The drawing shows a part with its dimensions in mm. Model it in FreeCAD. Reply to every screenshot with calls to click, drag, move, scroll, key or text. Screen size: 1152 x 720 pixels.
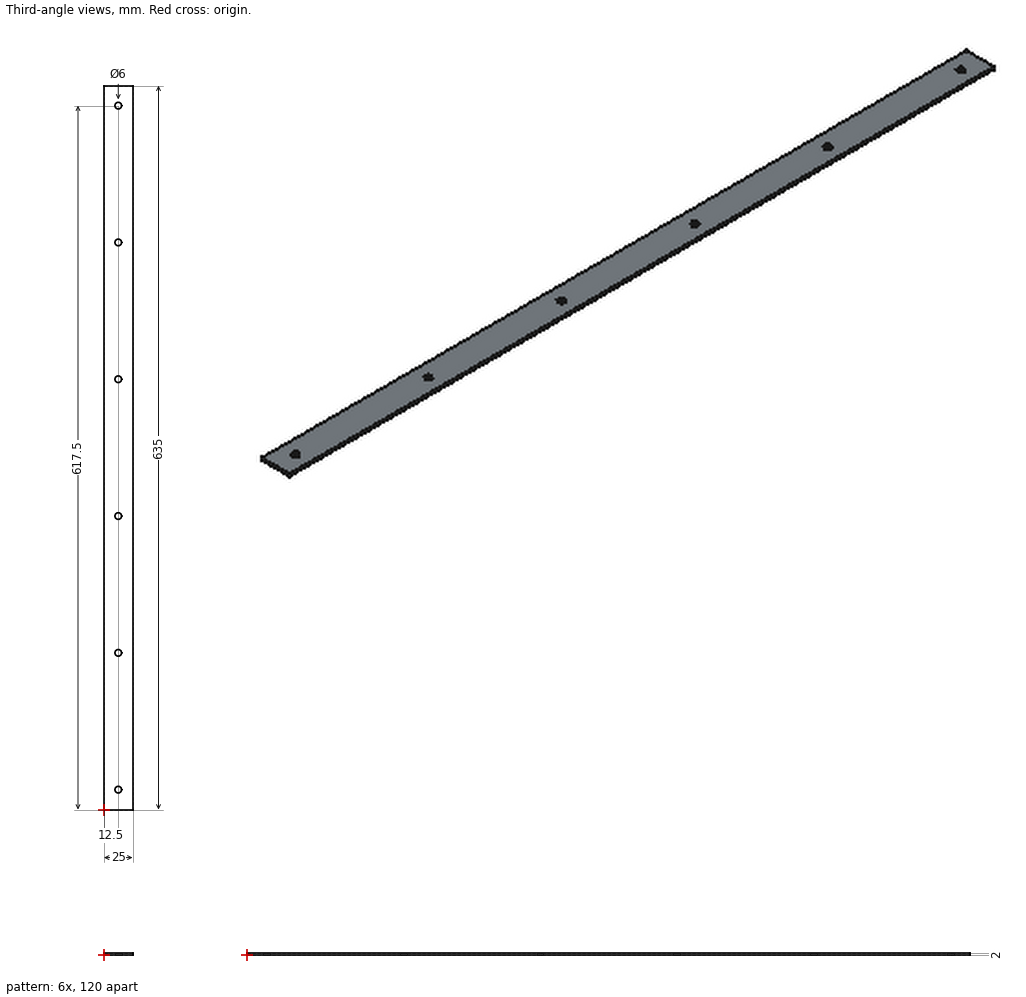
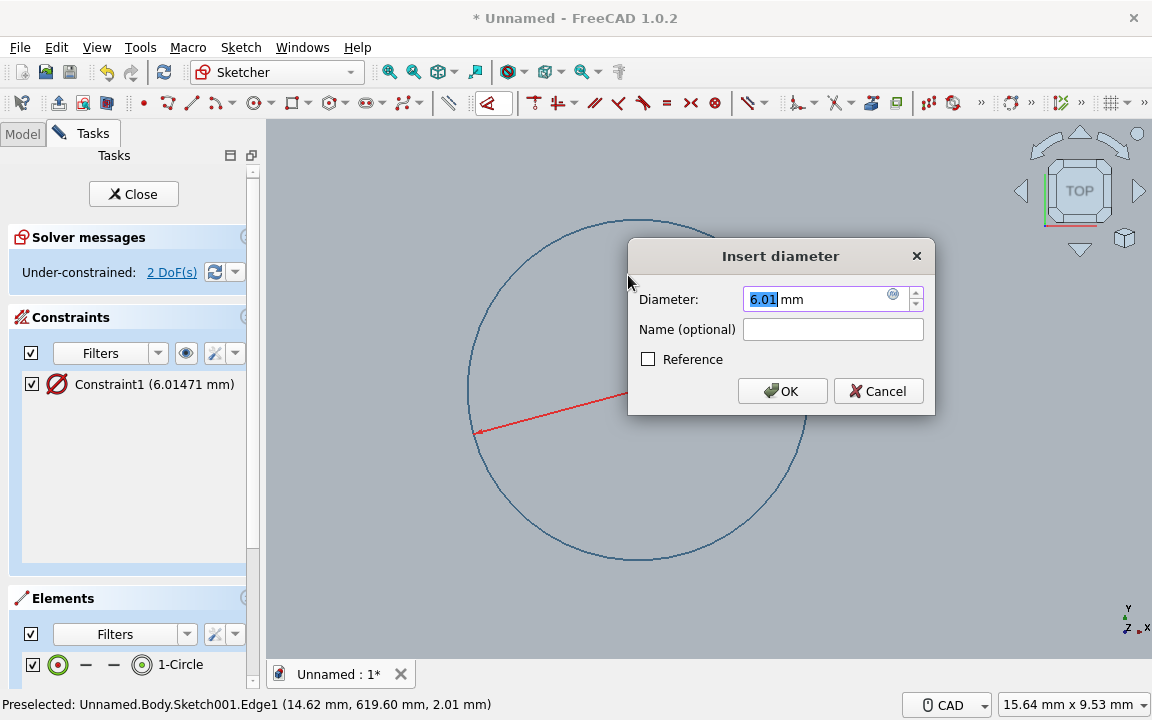
text(6)
key(Return)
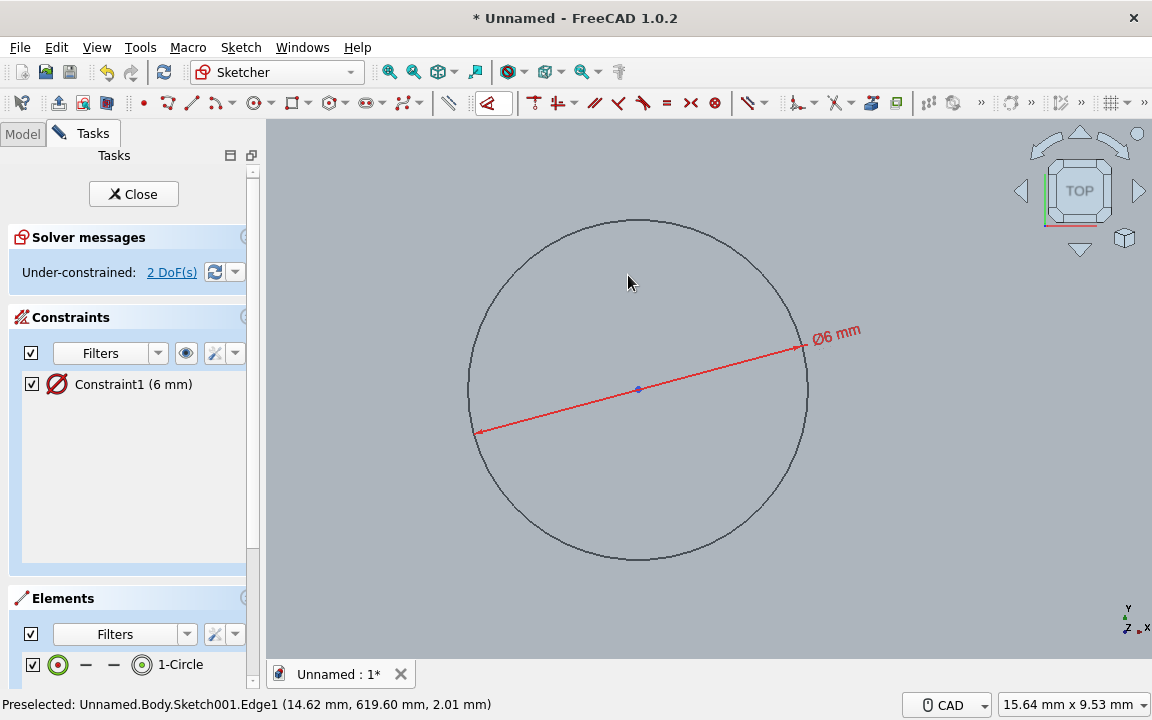
click(638, 390)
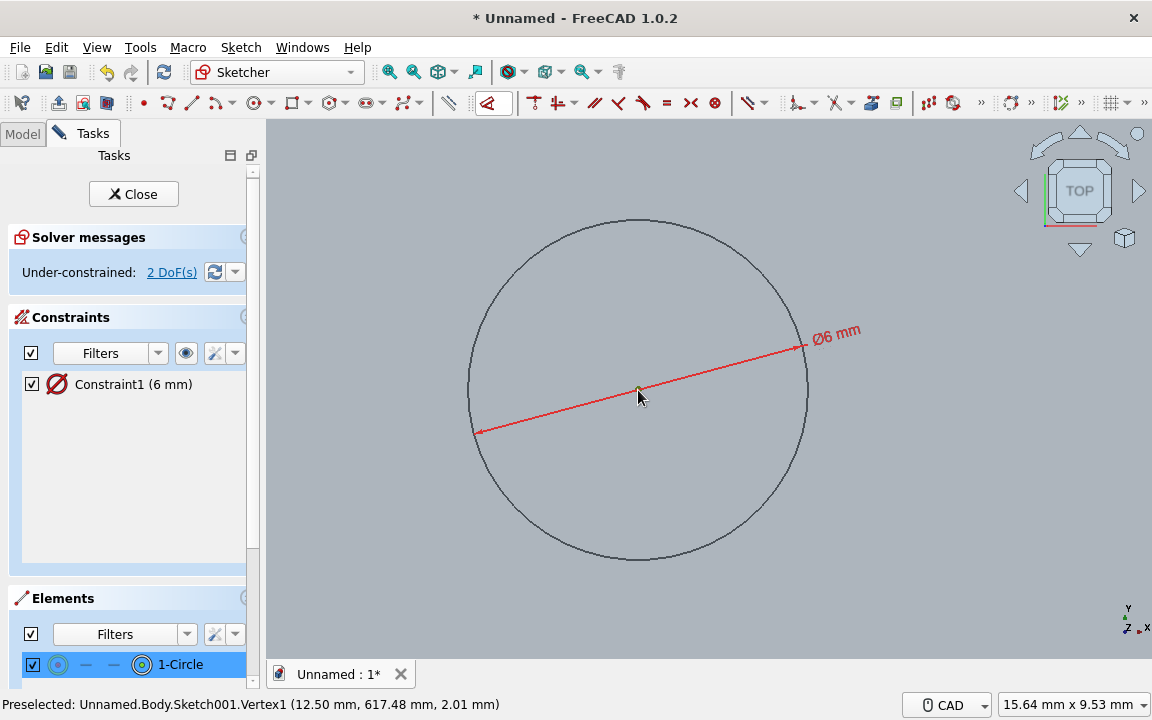
key(l)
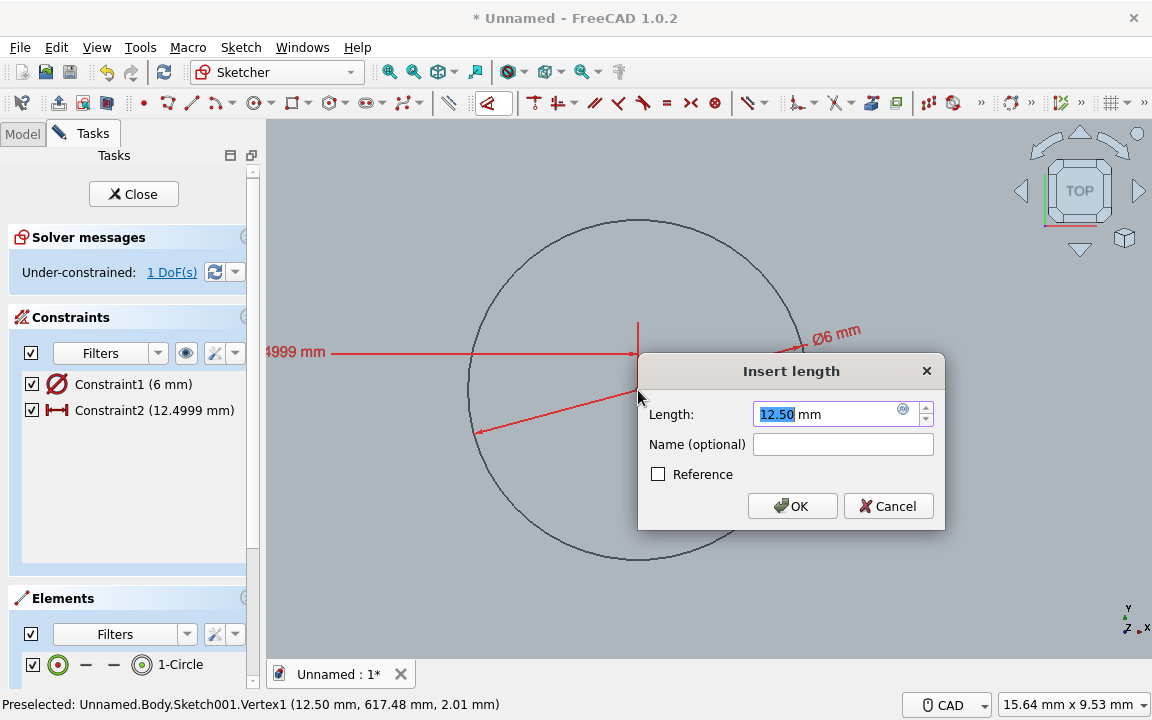
text(12.5)
key(Return)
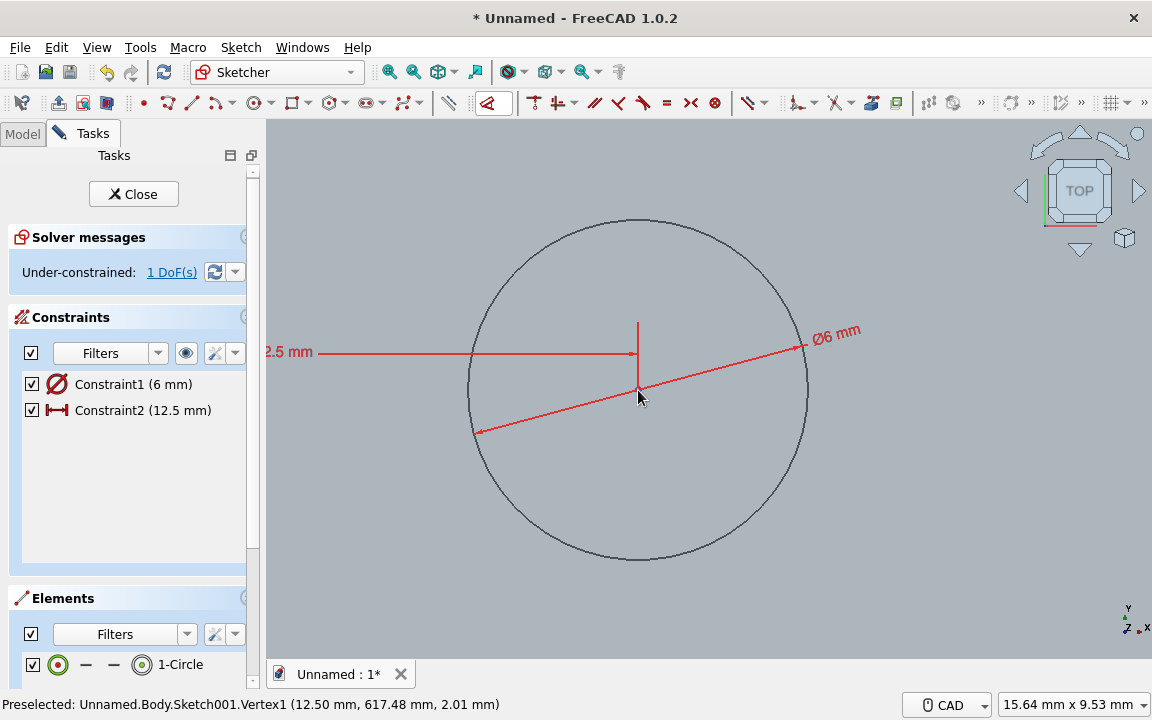
click(638, 390)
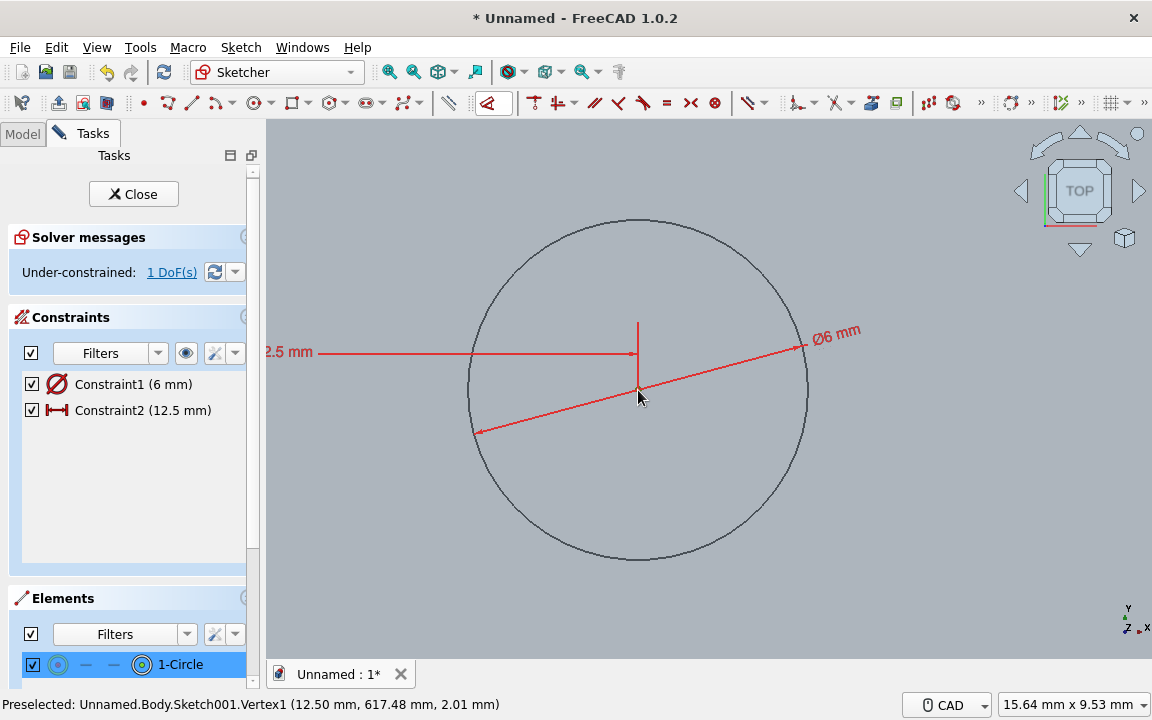
click(506, 104)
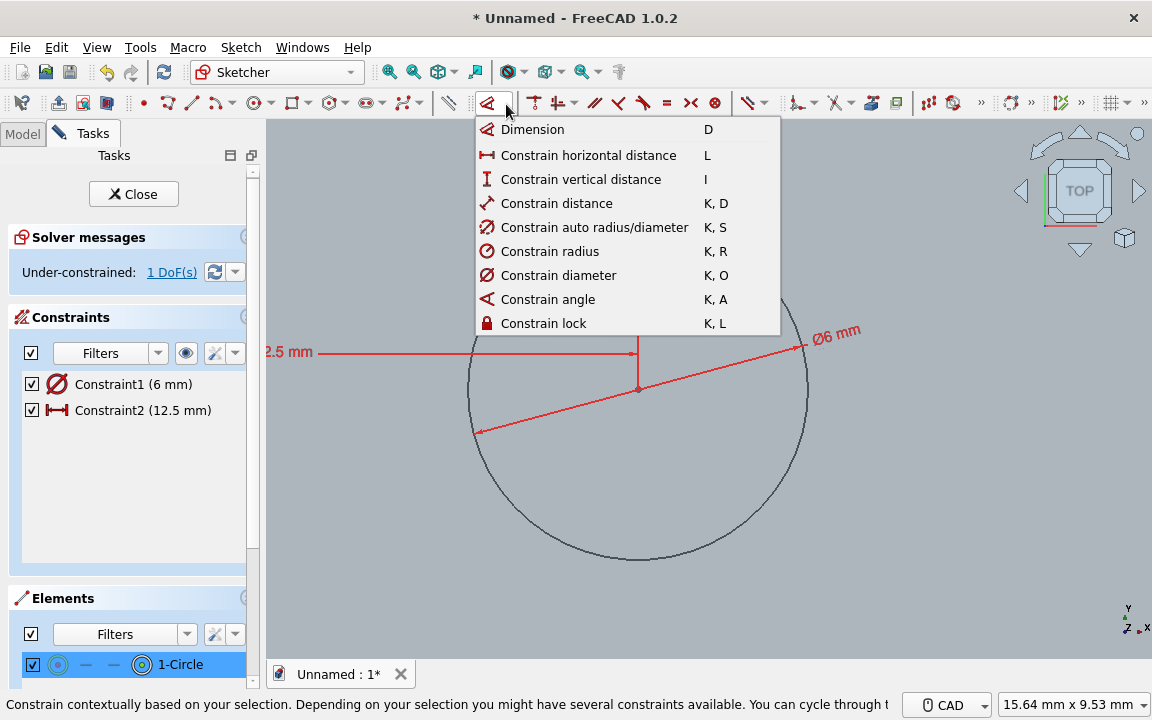
click(628, 179)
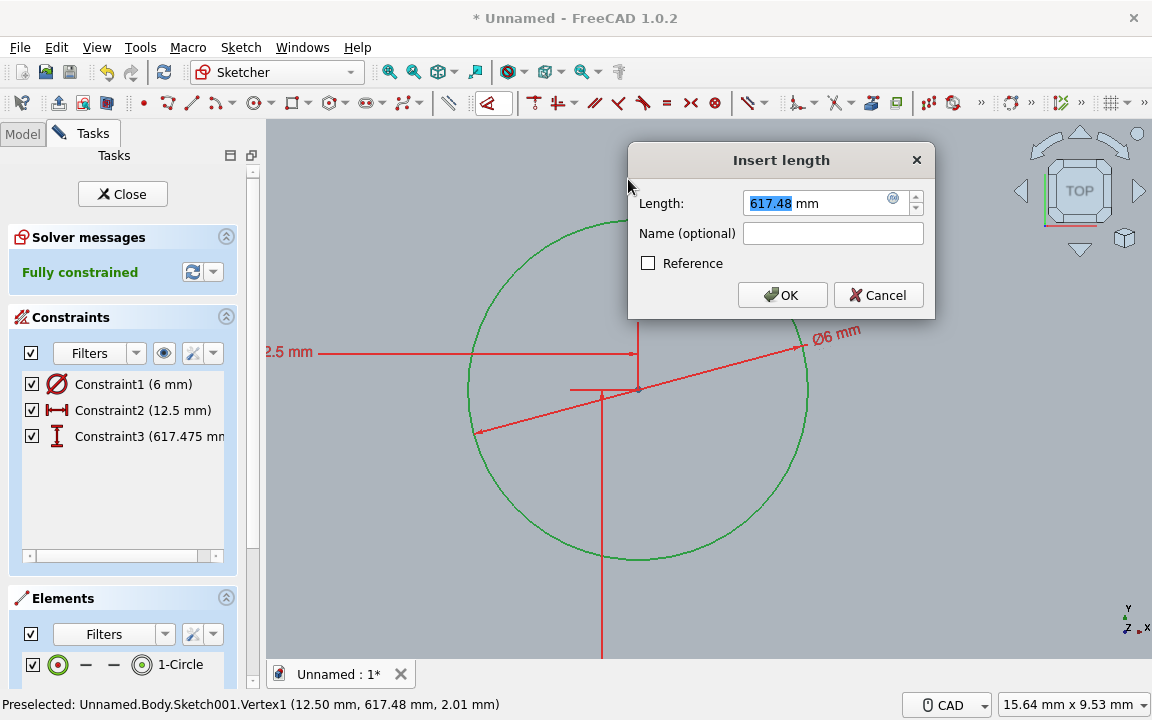
text(617.5)
key(Return)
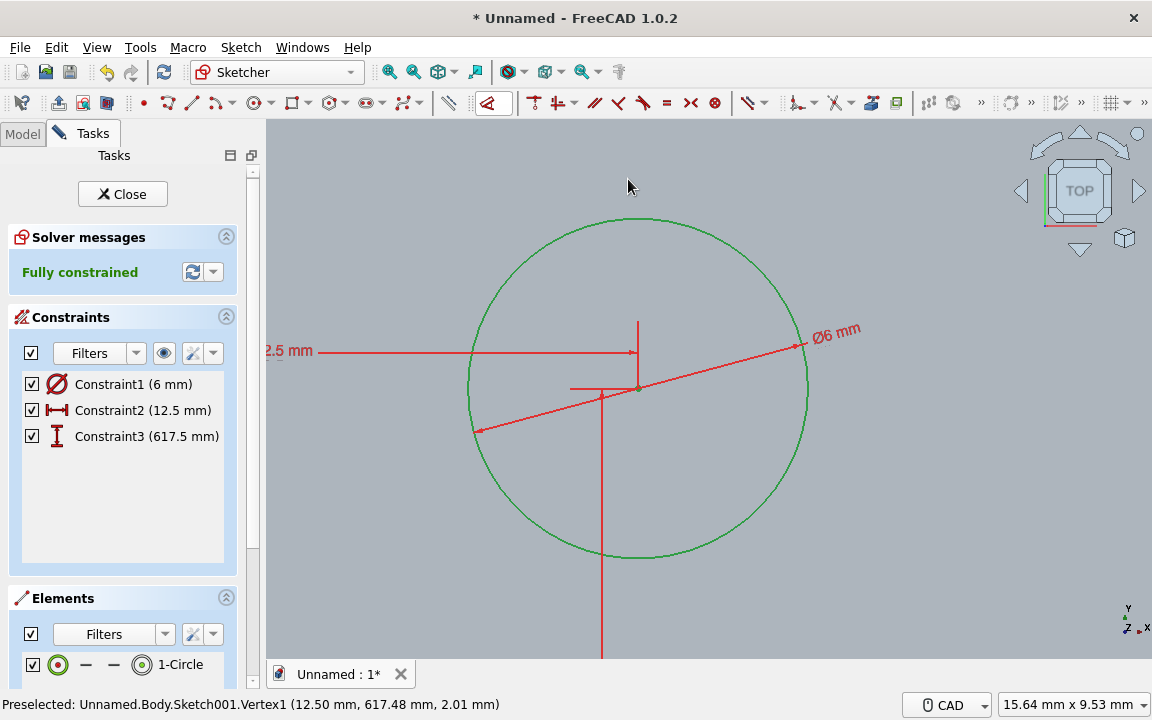
click(123, 194)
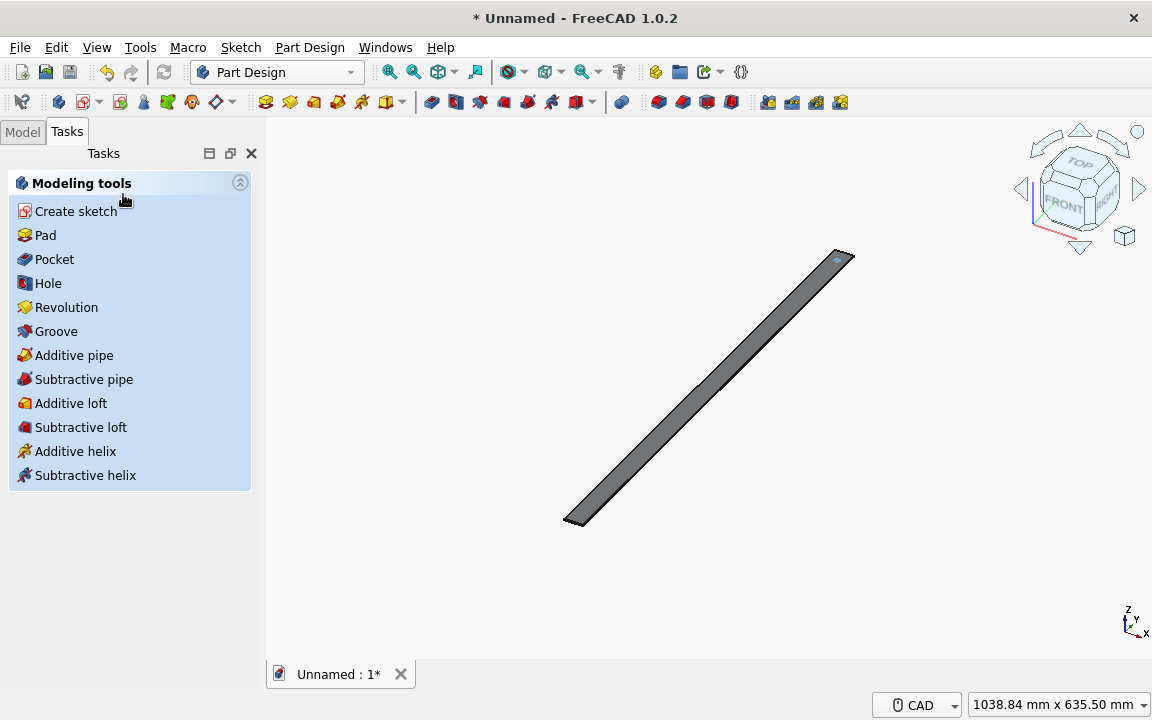
click(432, 102)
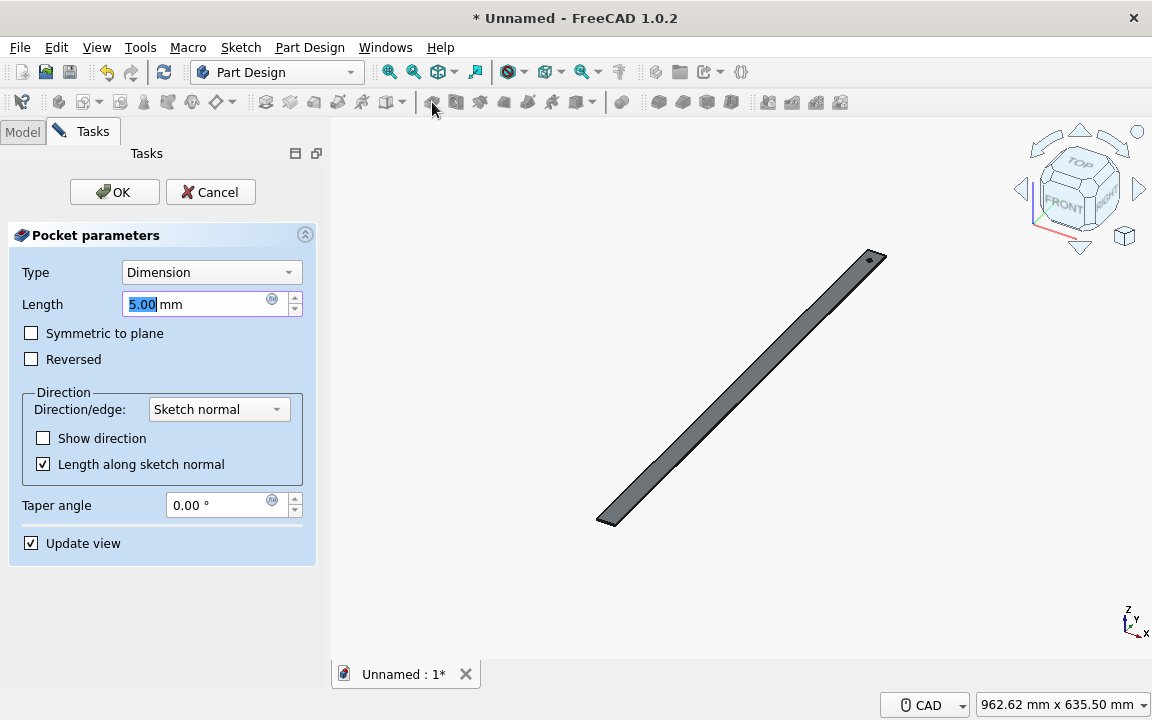
click(212, 272)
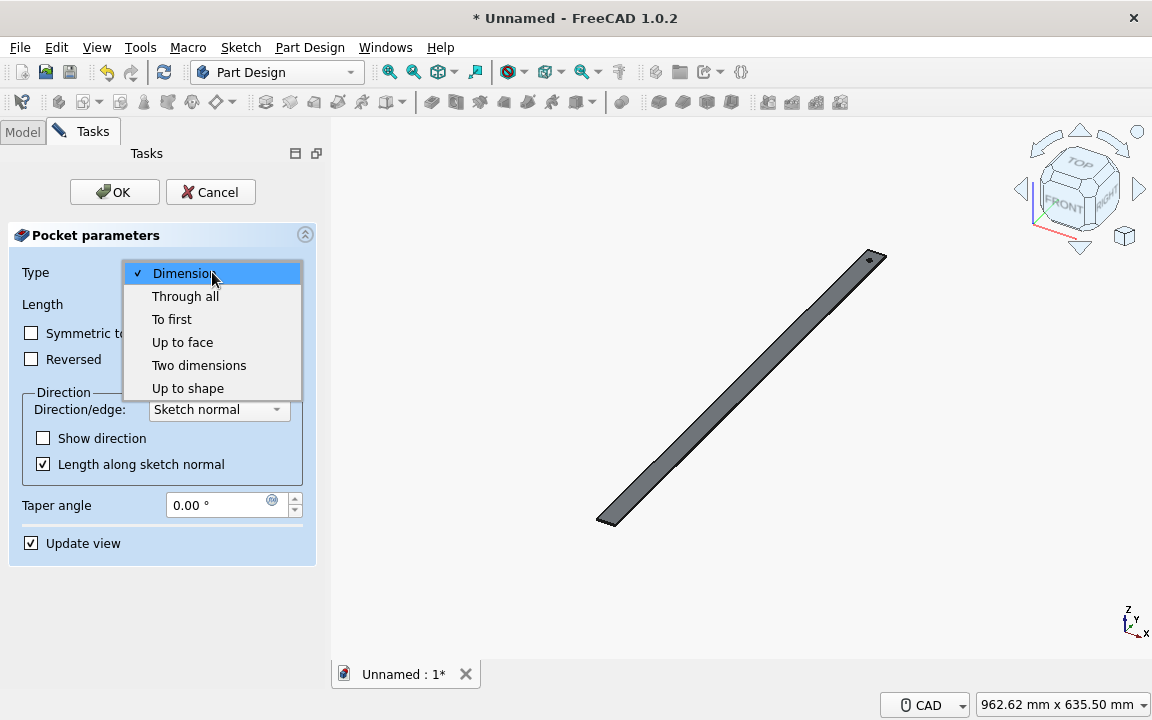
click(212, 296)